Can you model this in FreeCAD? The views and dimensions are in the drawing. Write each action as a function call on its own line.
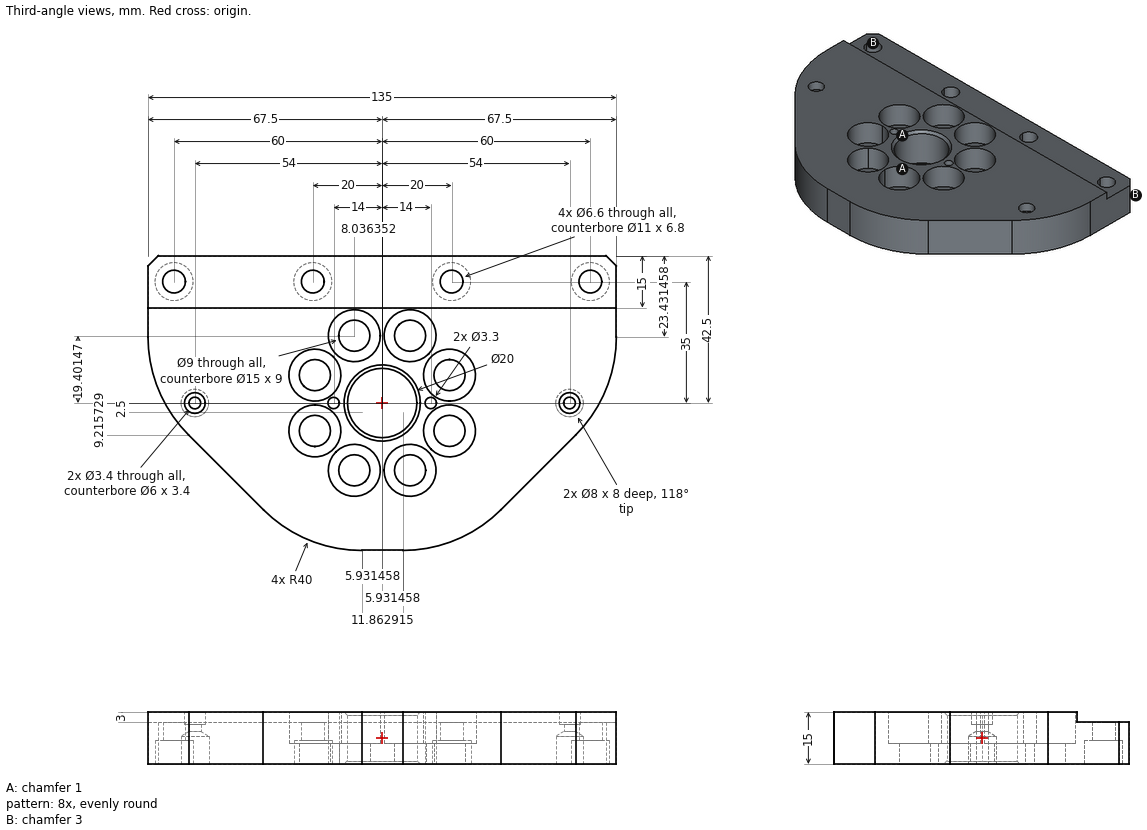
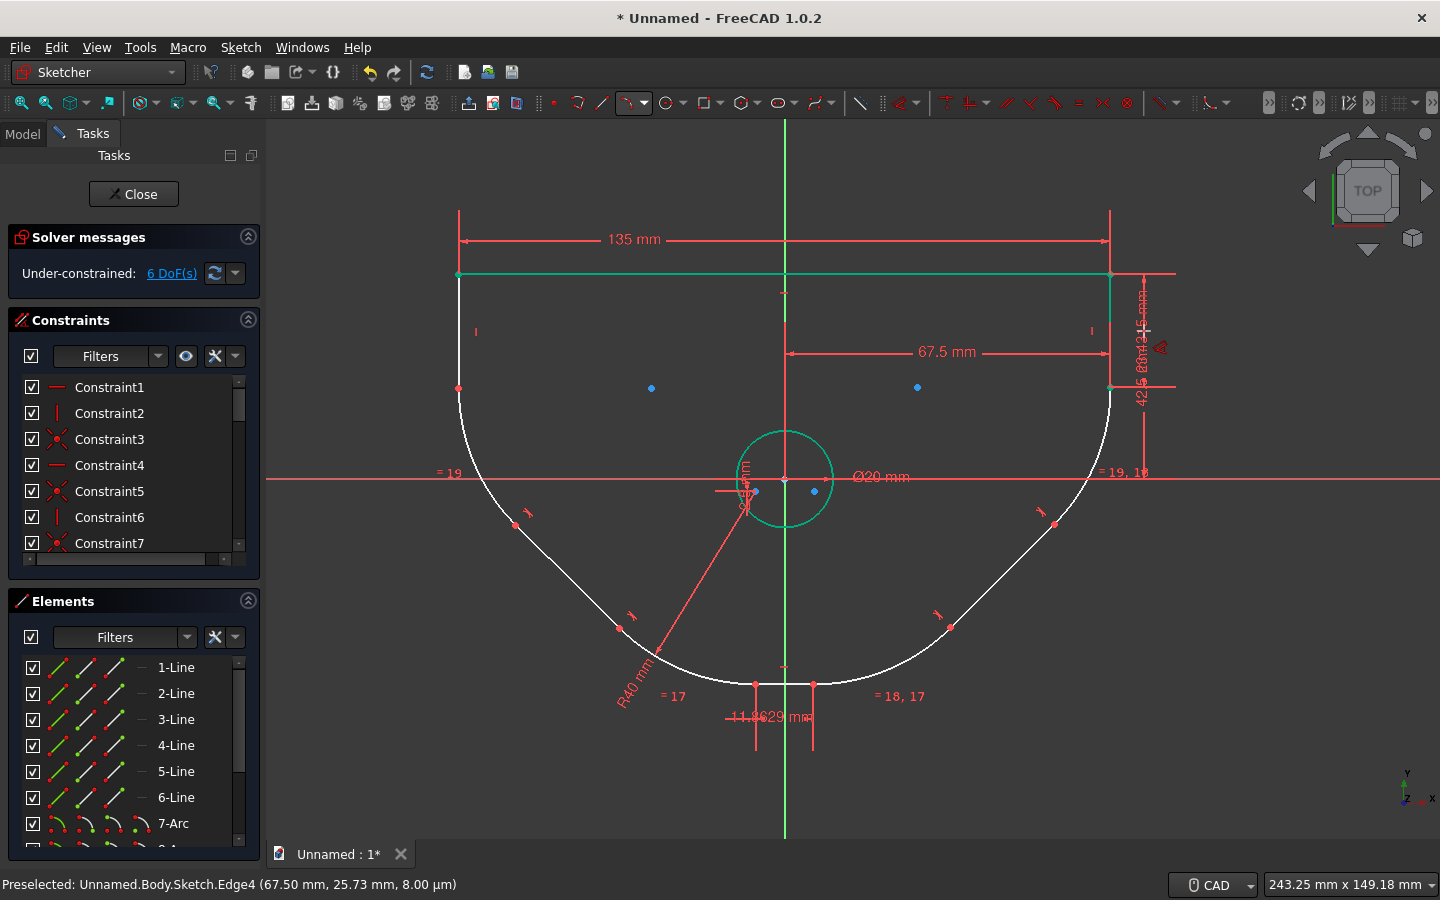
click(459, 308)
click(425, 331)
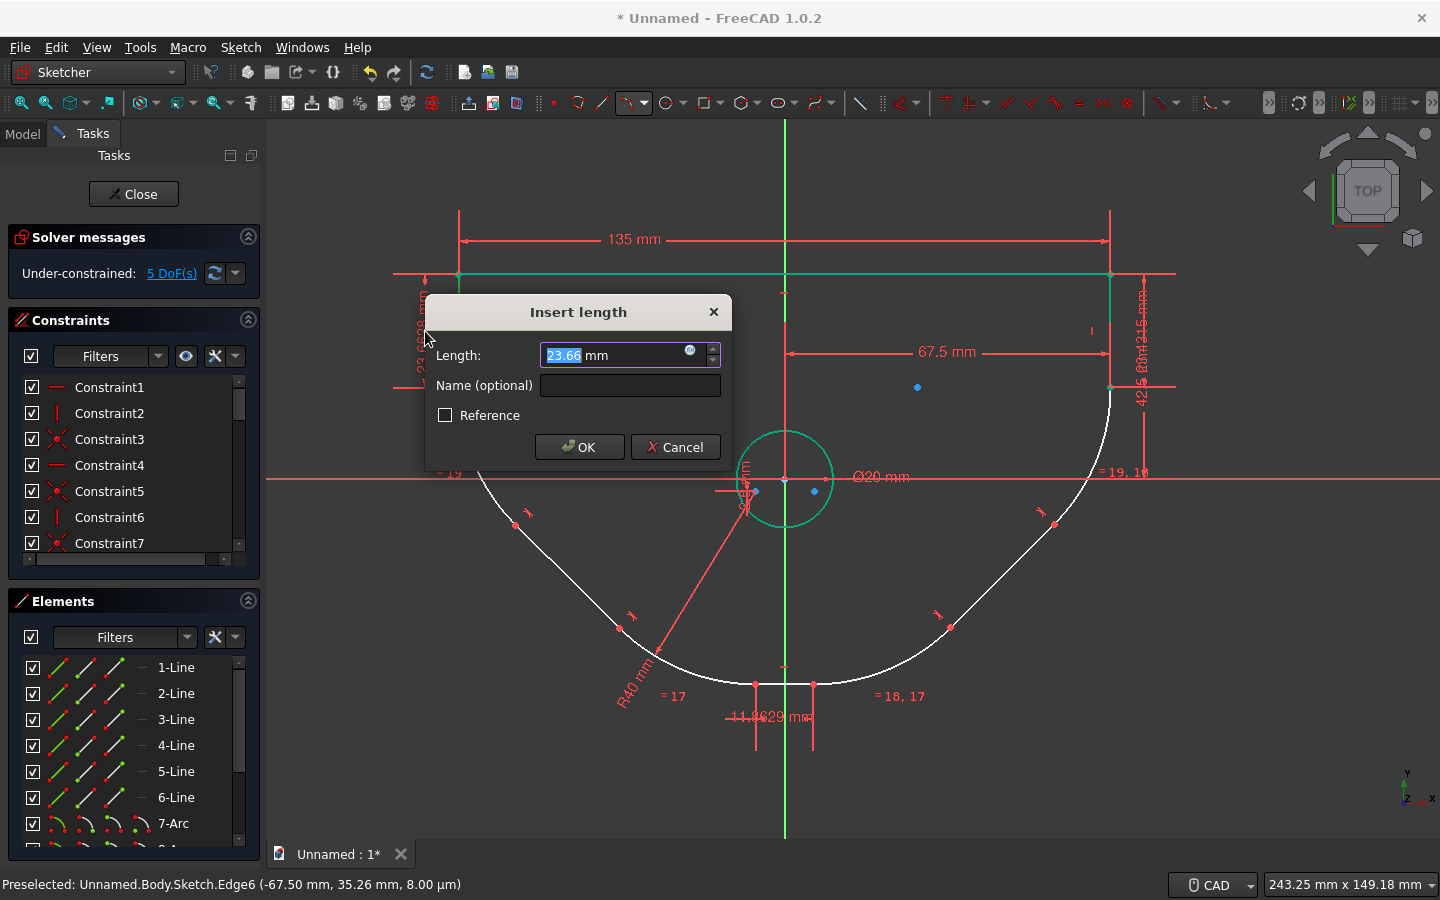
text(23.431458)
key(Return)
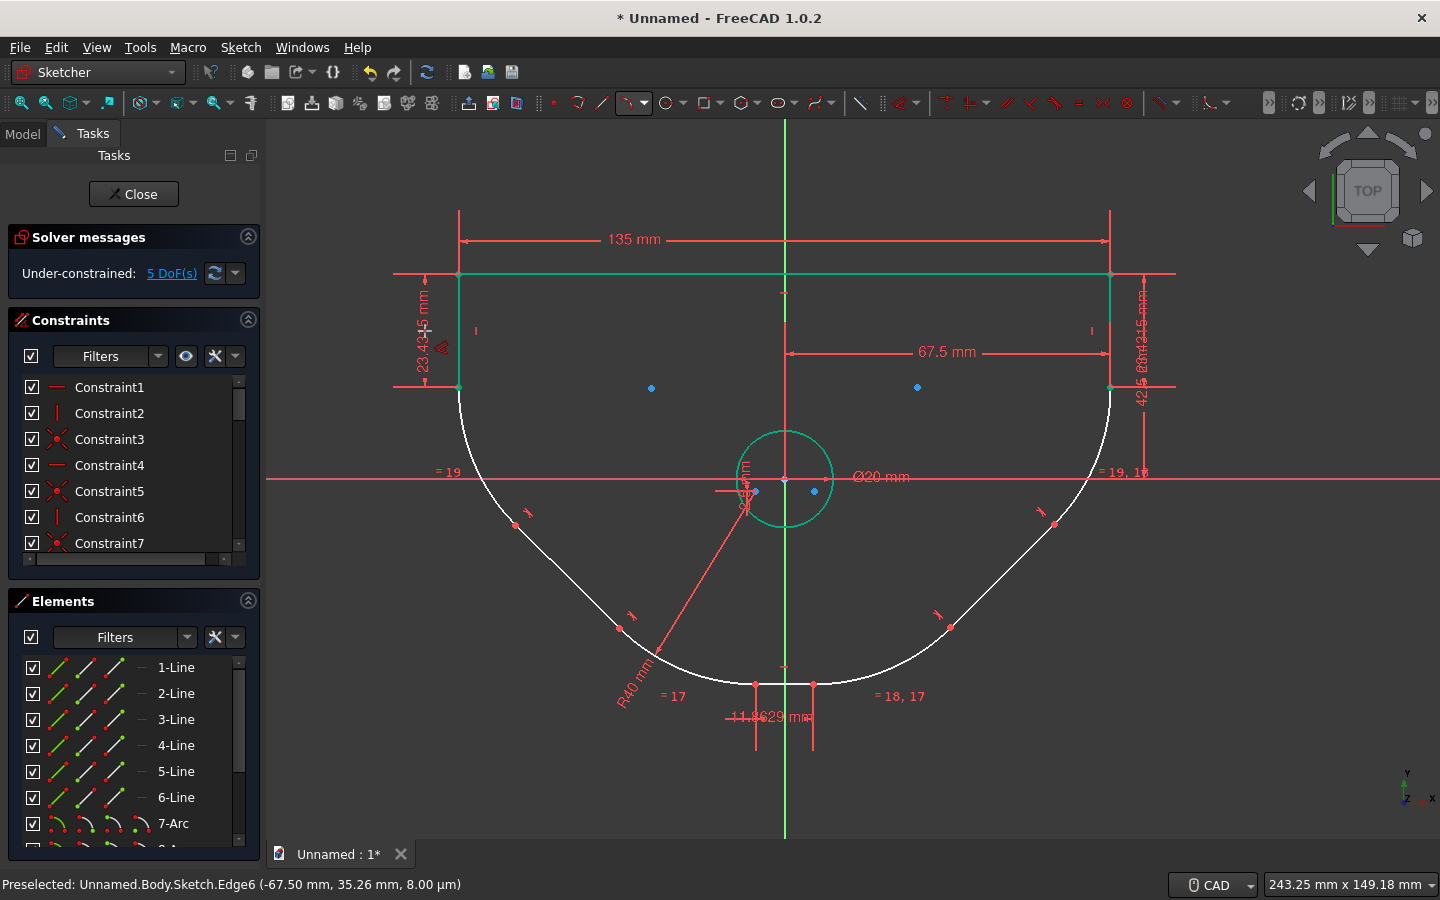
click(516, 525)
click(482, 513)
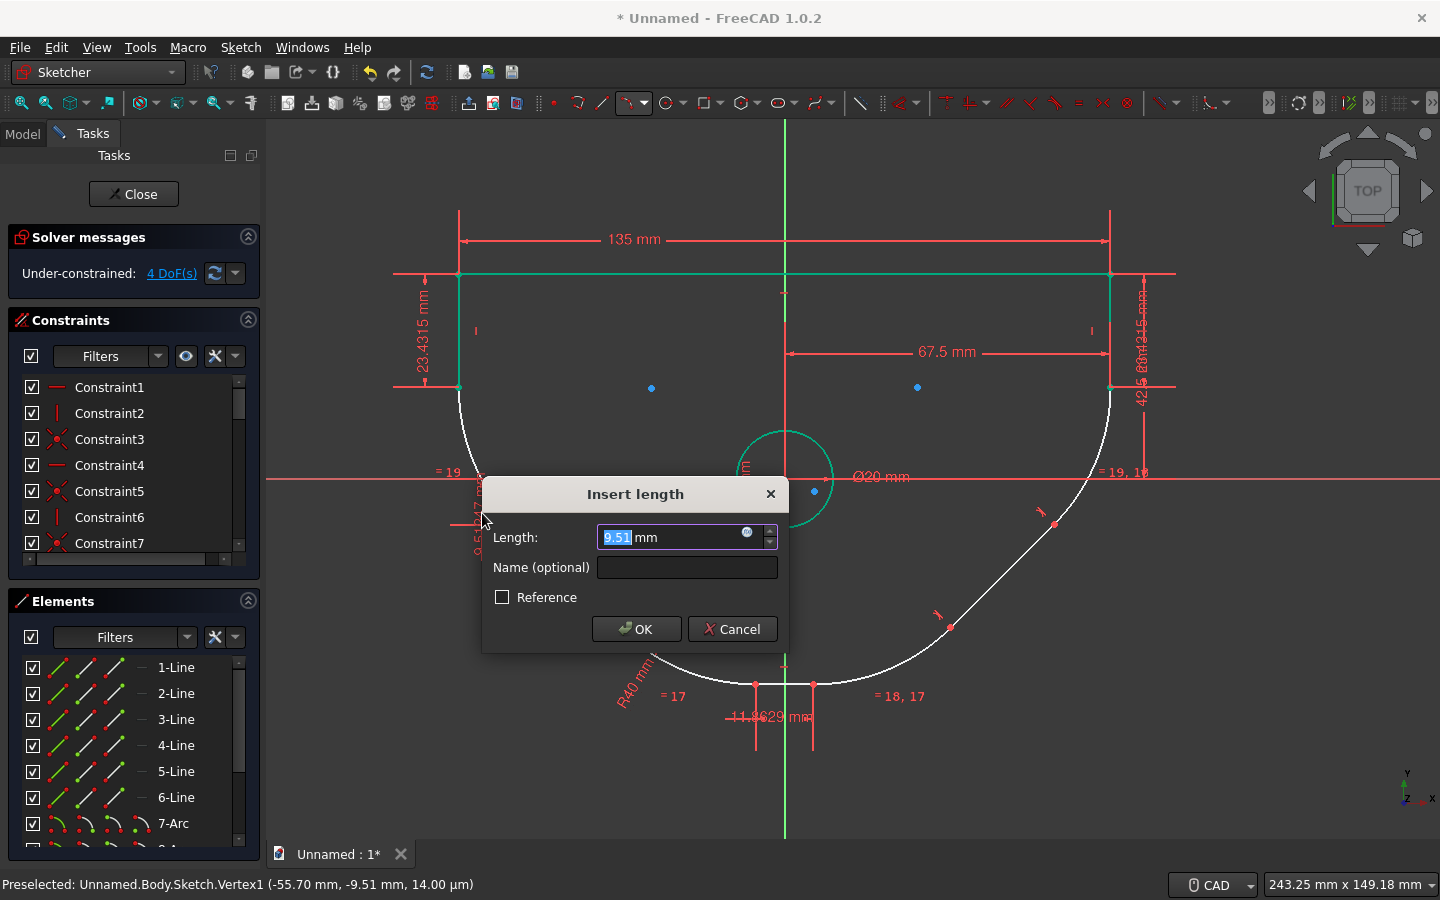
text(9.215729)
key(Return)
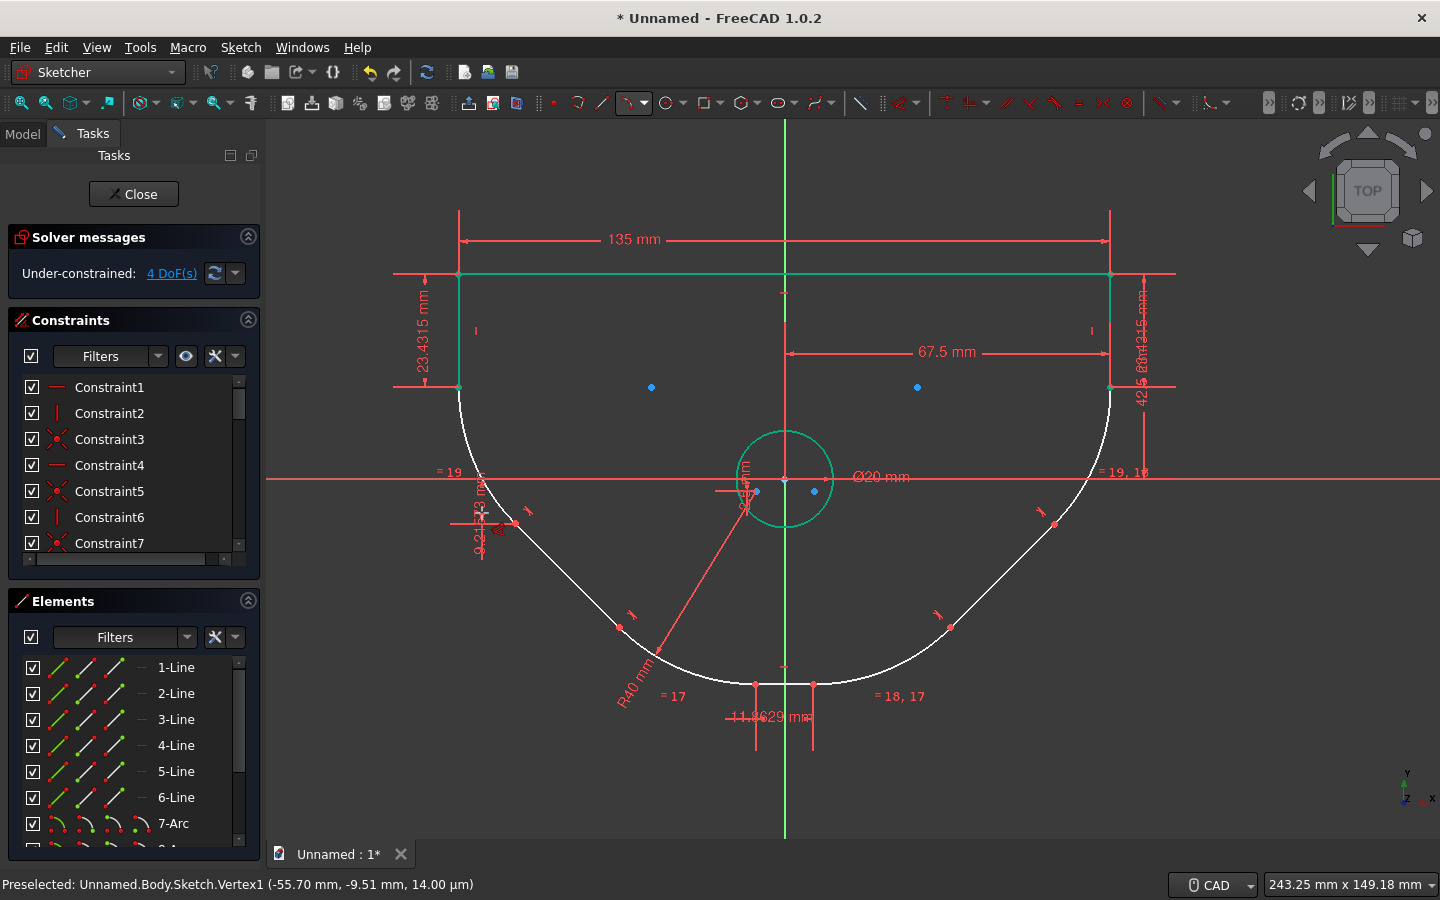
scroll(756, 684, up, 2)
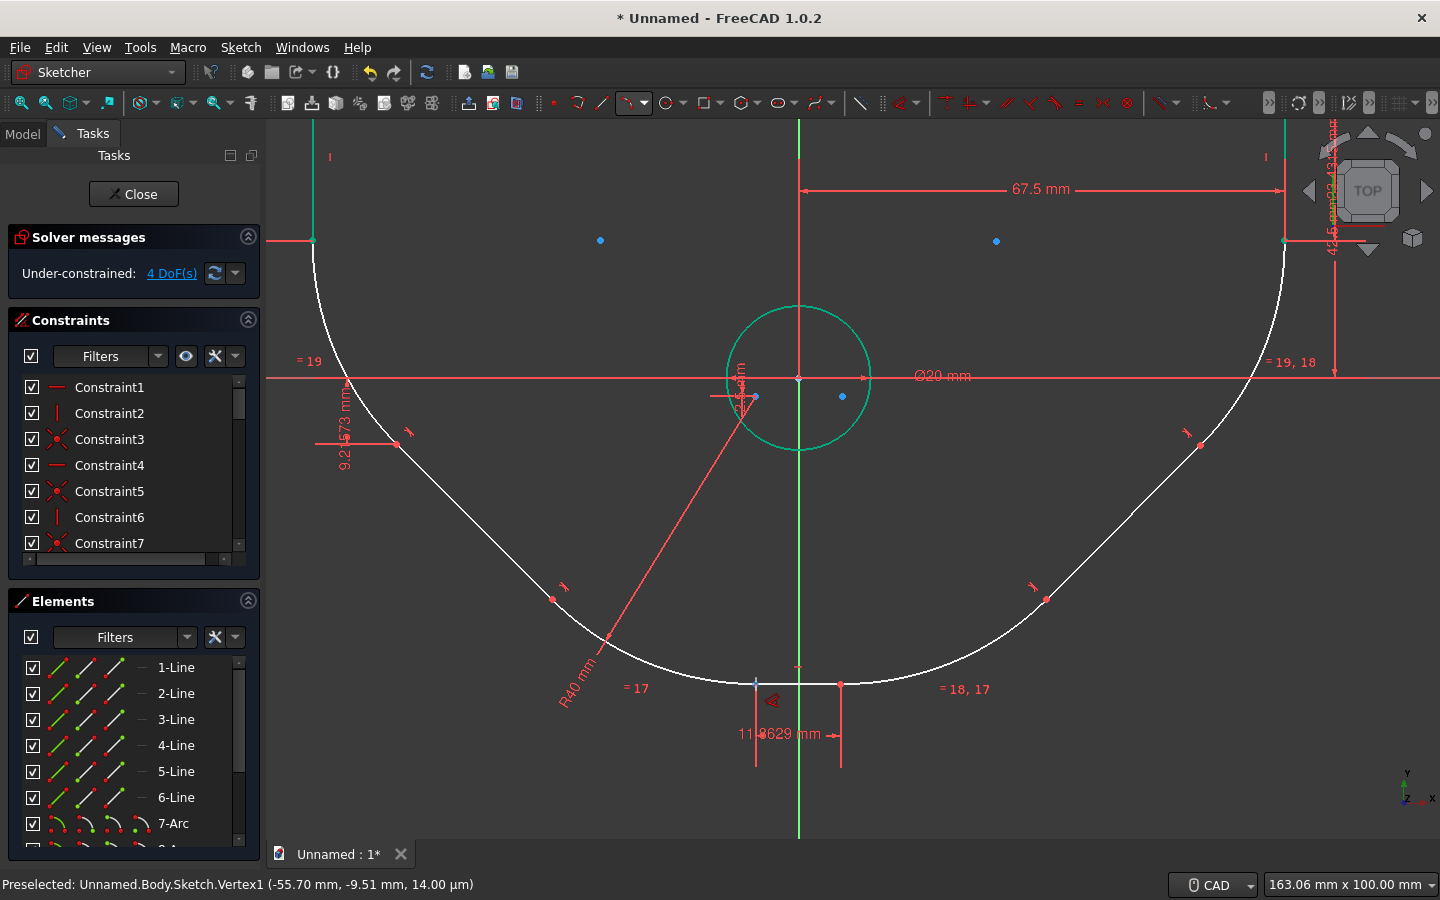
click(756, 684)
click(777, 344)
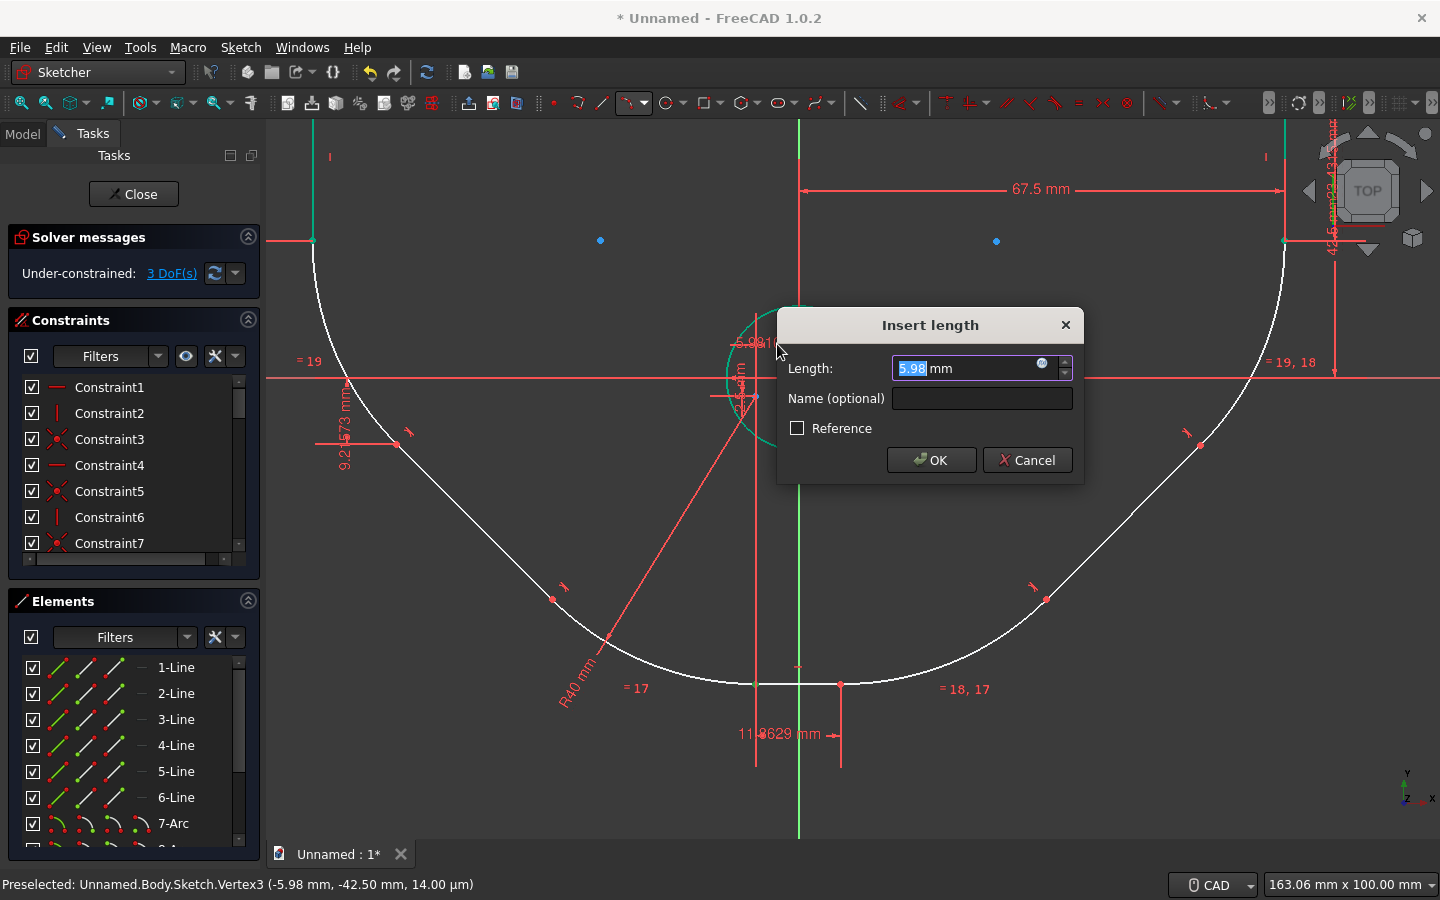
text(5.931458)
key(Return)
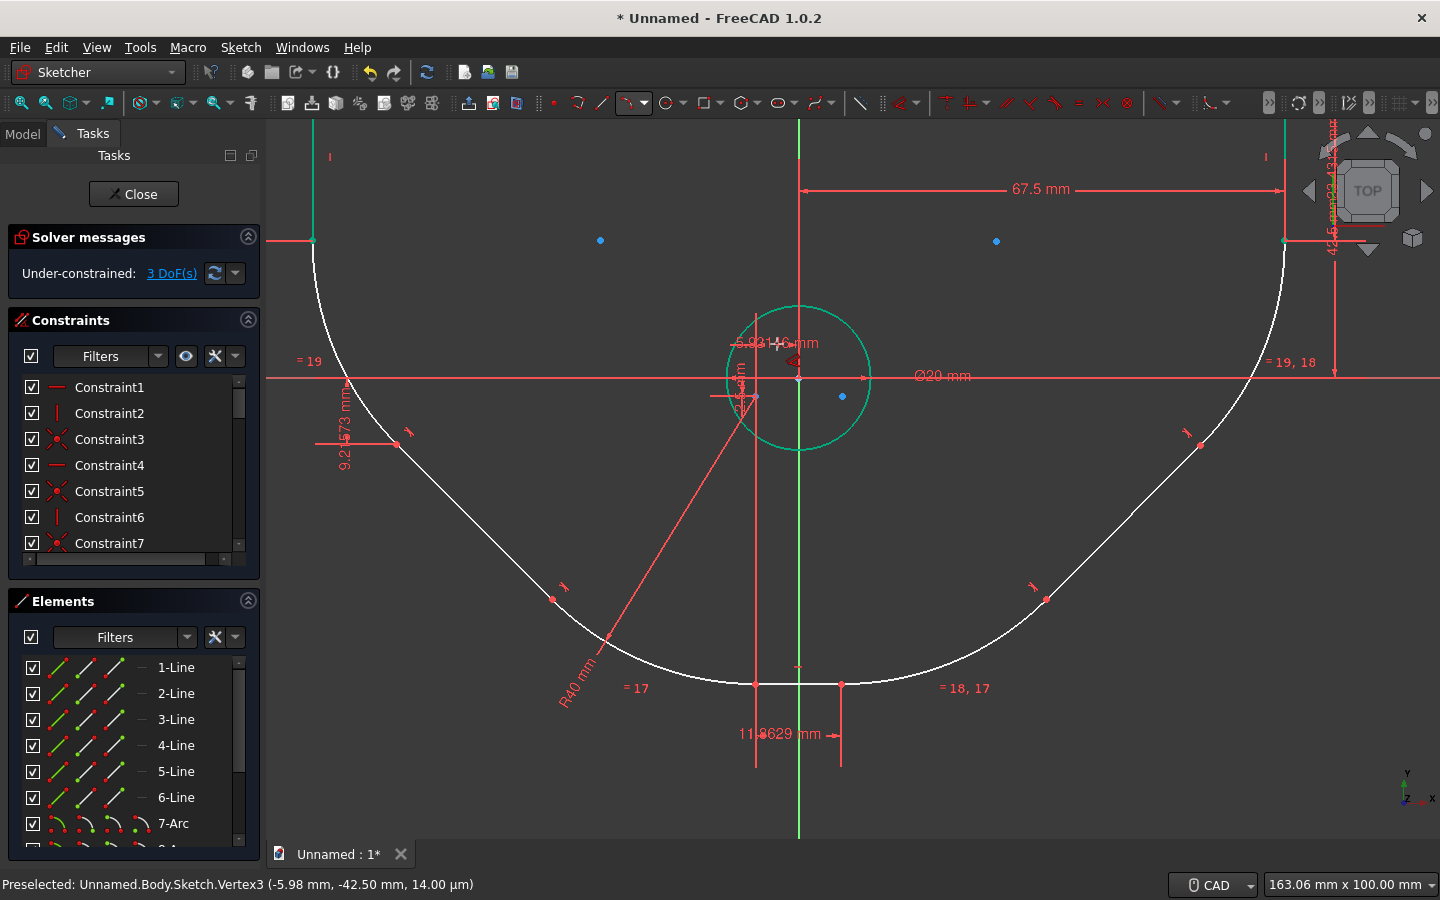
click(1200, 445)
click(1234, 427)